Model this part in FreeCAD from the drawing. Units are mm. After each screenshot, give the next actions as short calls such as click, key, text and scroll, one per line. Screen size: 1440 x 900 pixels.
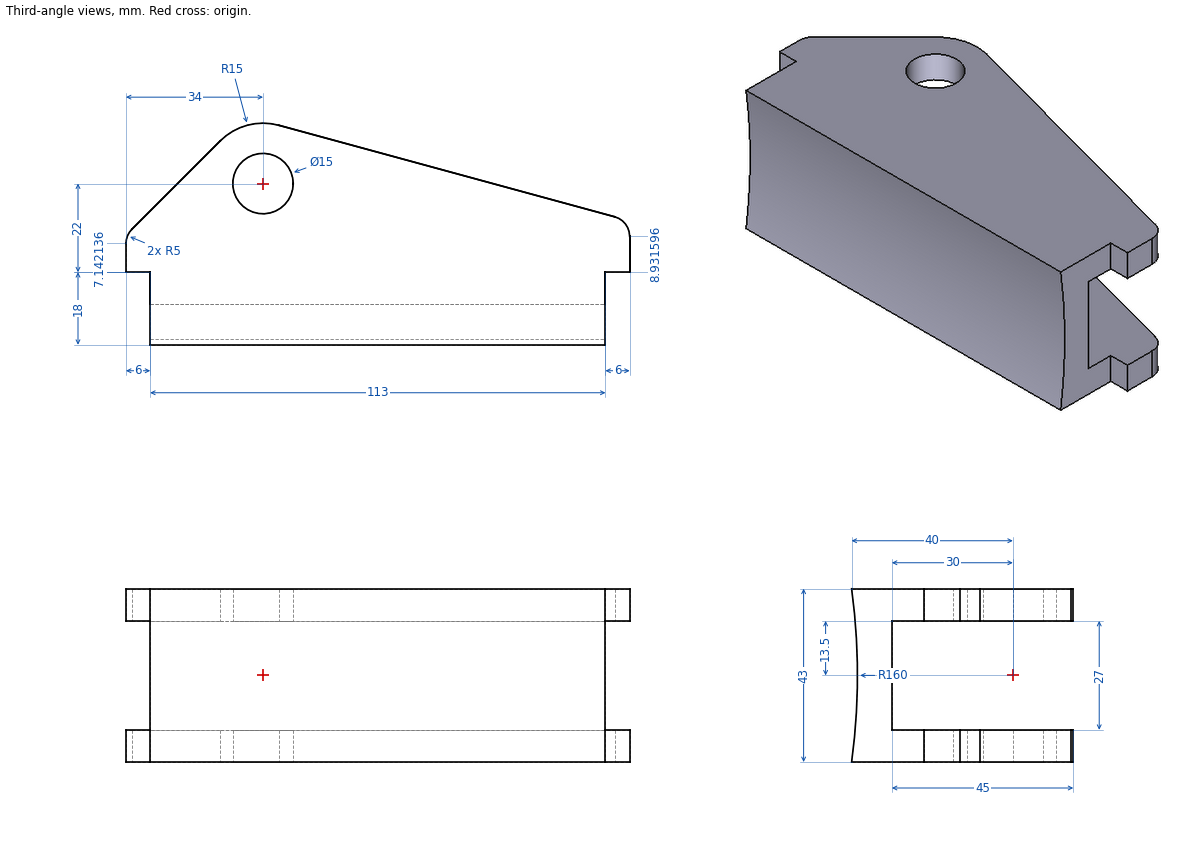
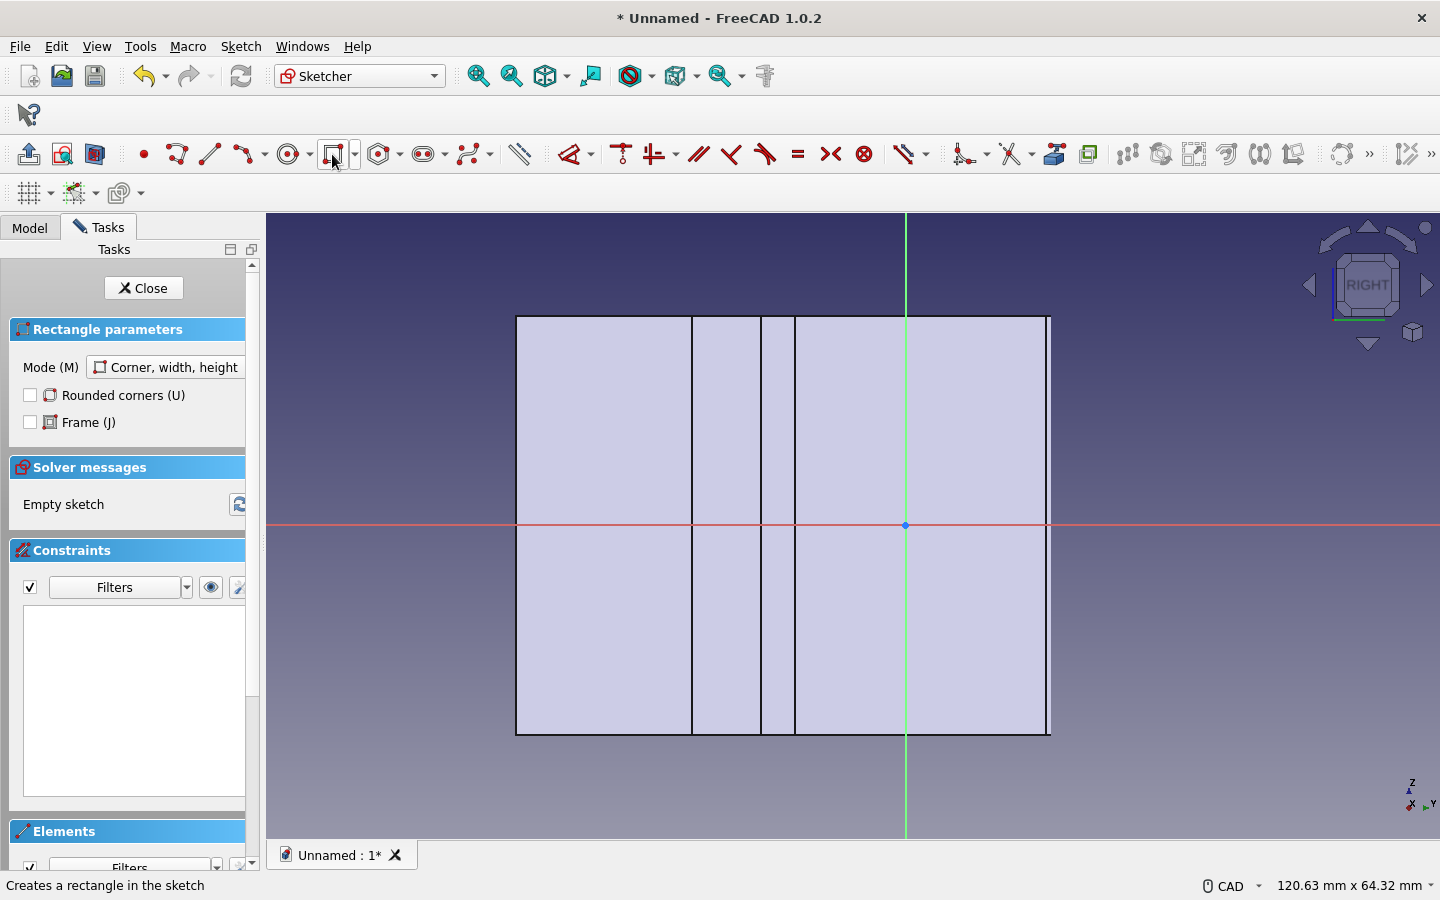
click(614, 394)
move(1052, 657)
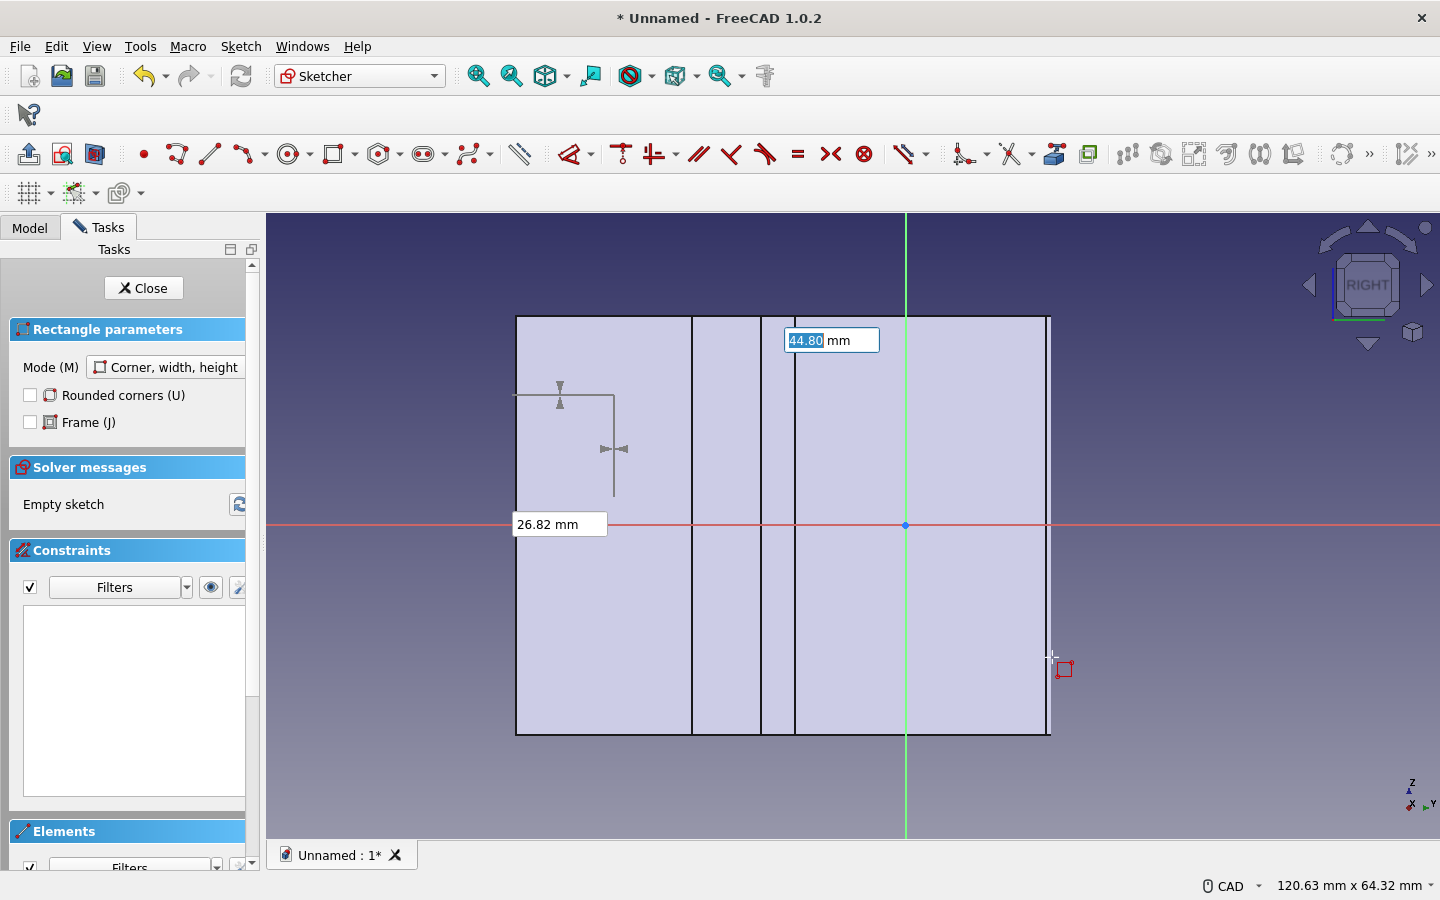
text(45)
key(Tab)
text(27)
key(Return)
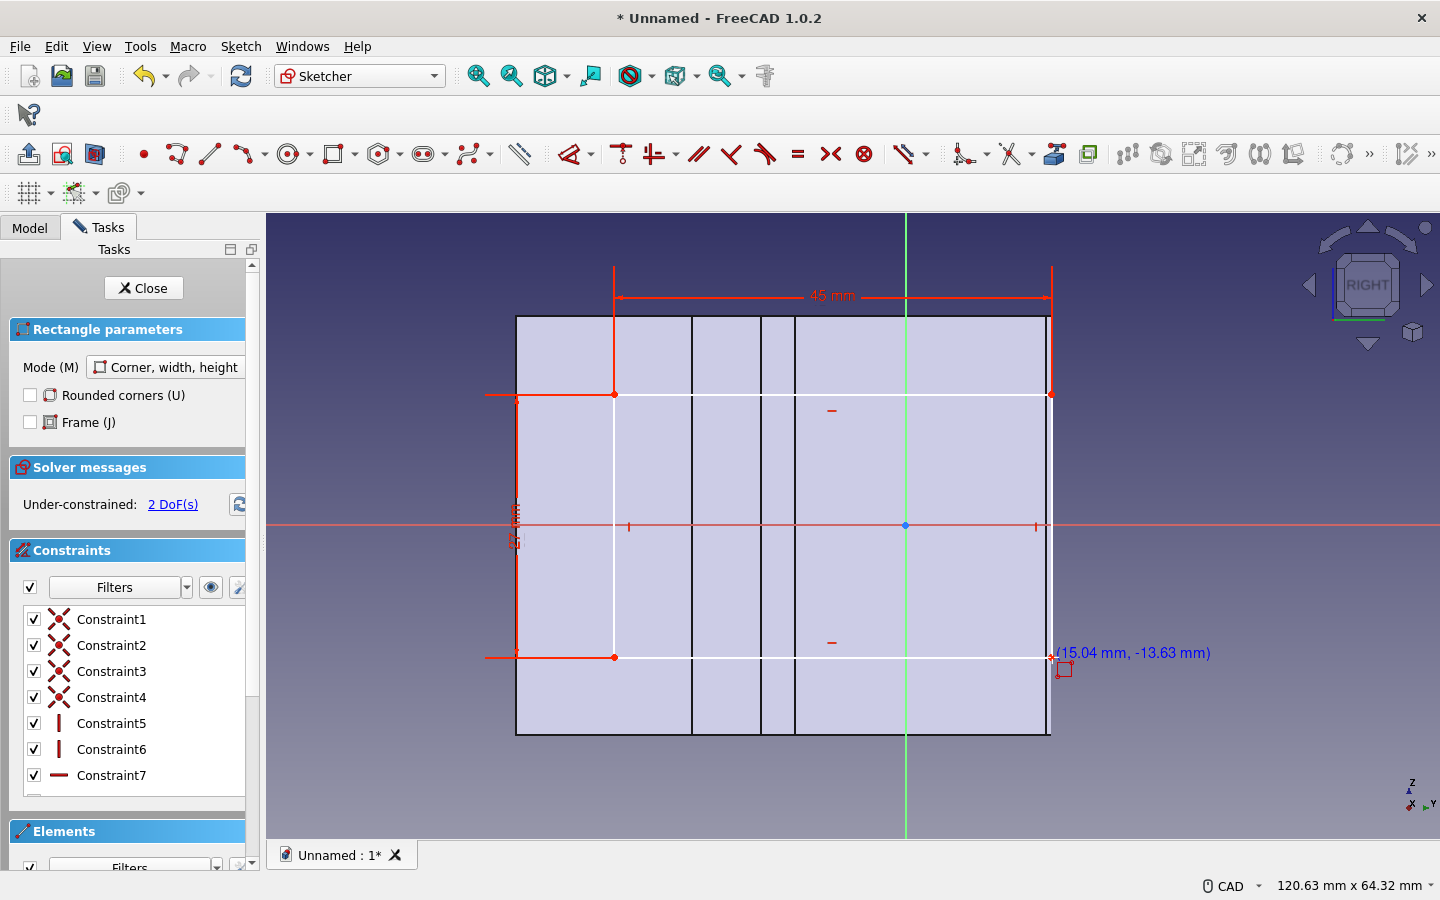
click(210, 154)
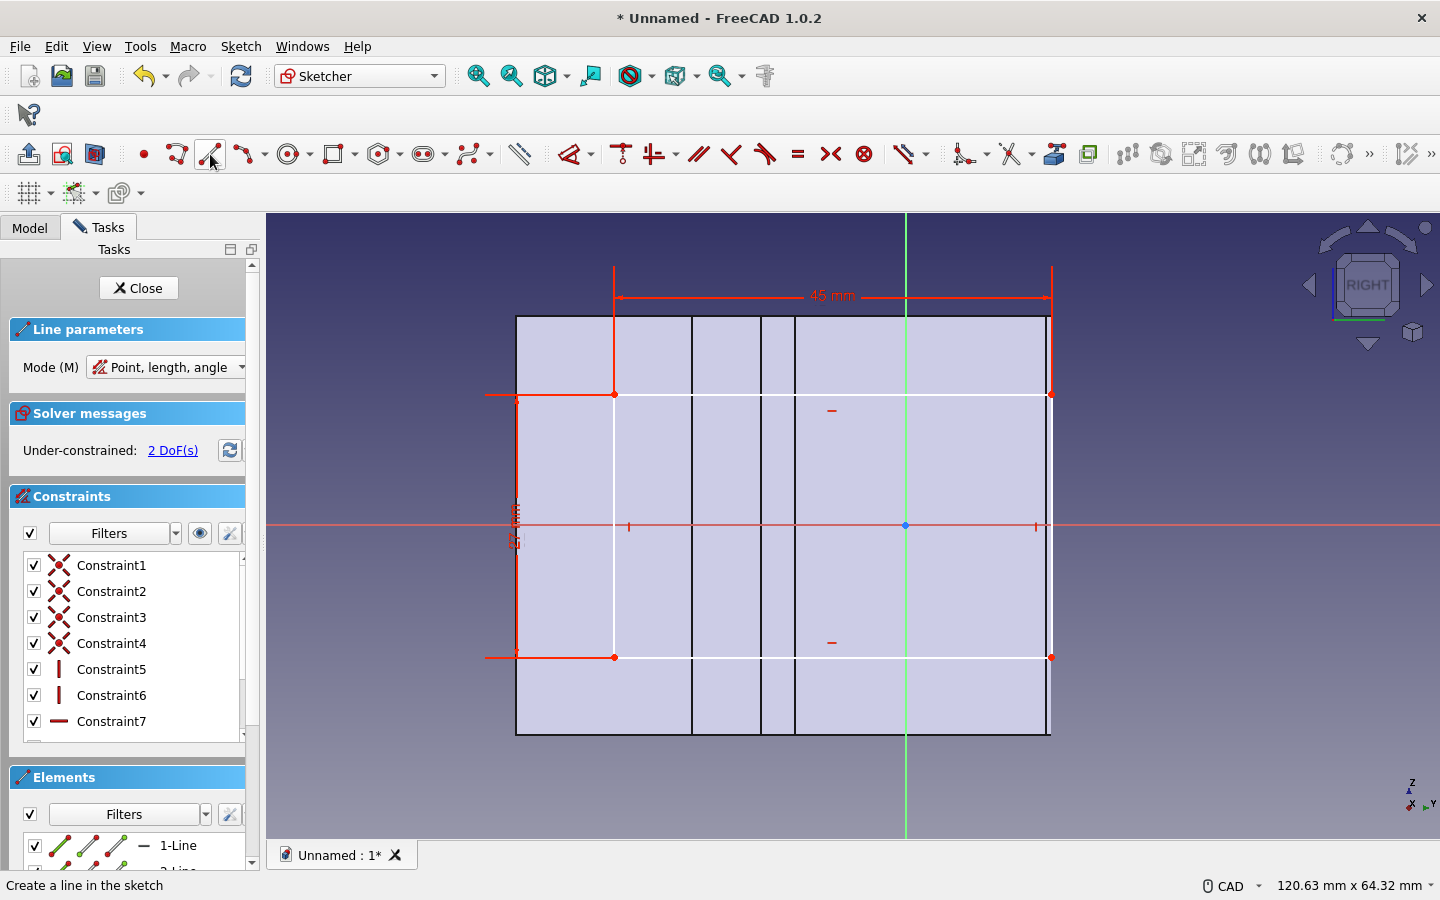
click(516, 316)
click(516, 735)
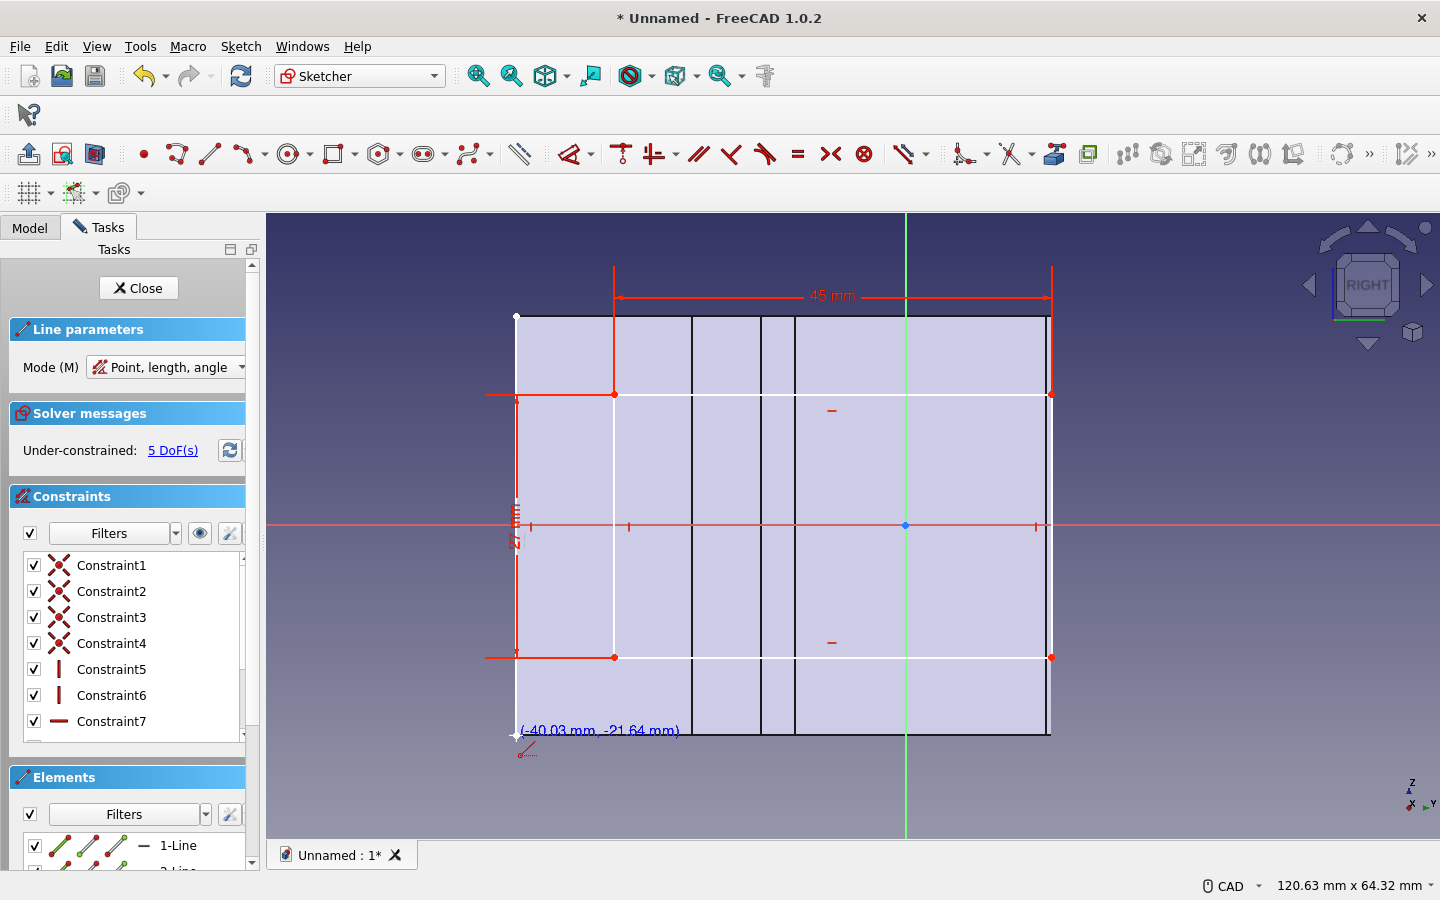
click(242, 154)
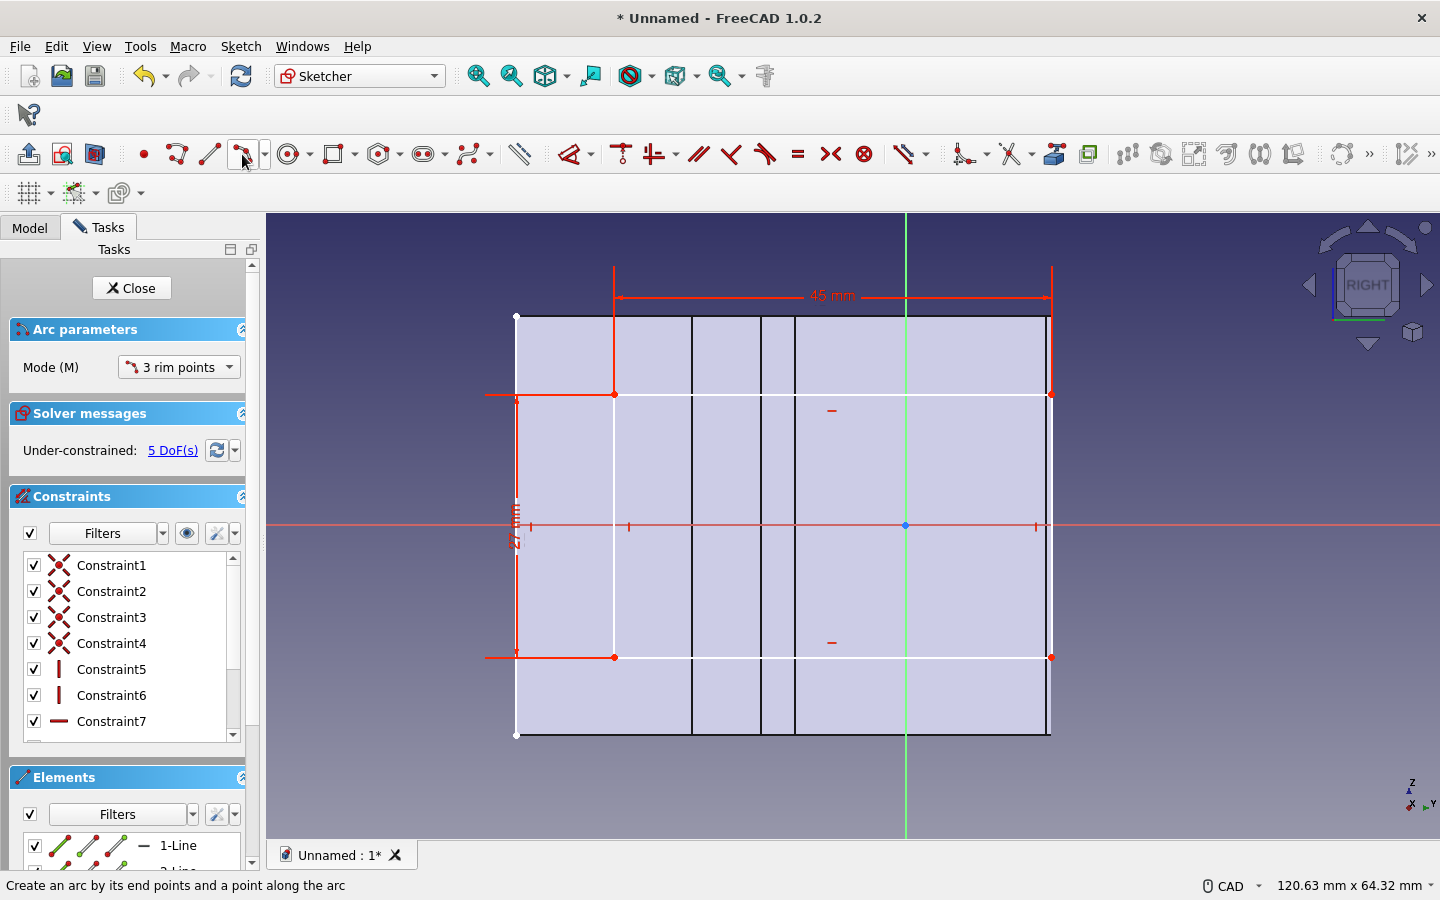
click(516, 736)
click(516, 317)
click(530, 567)
key(Escape)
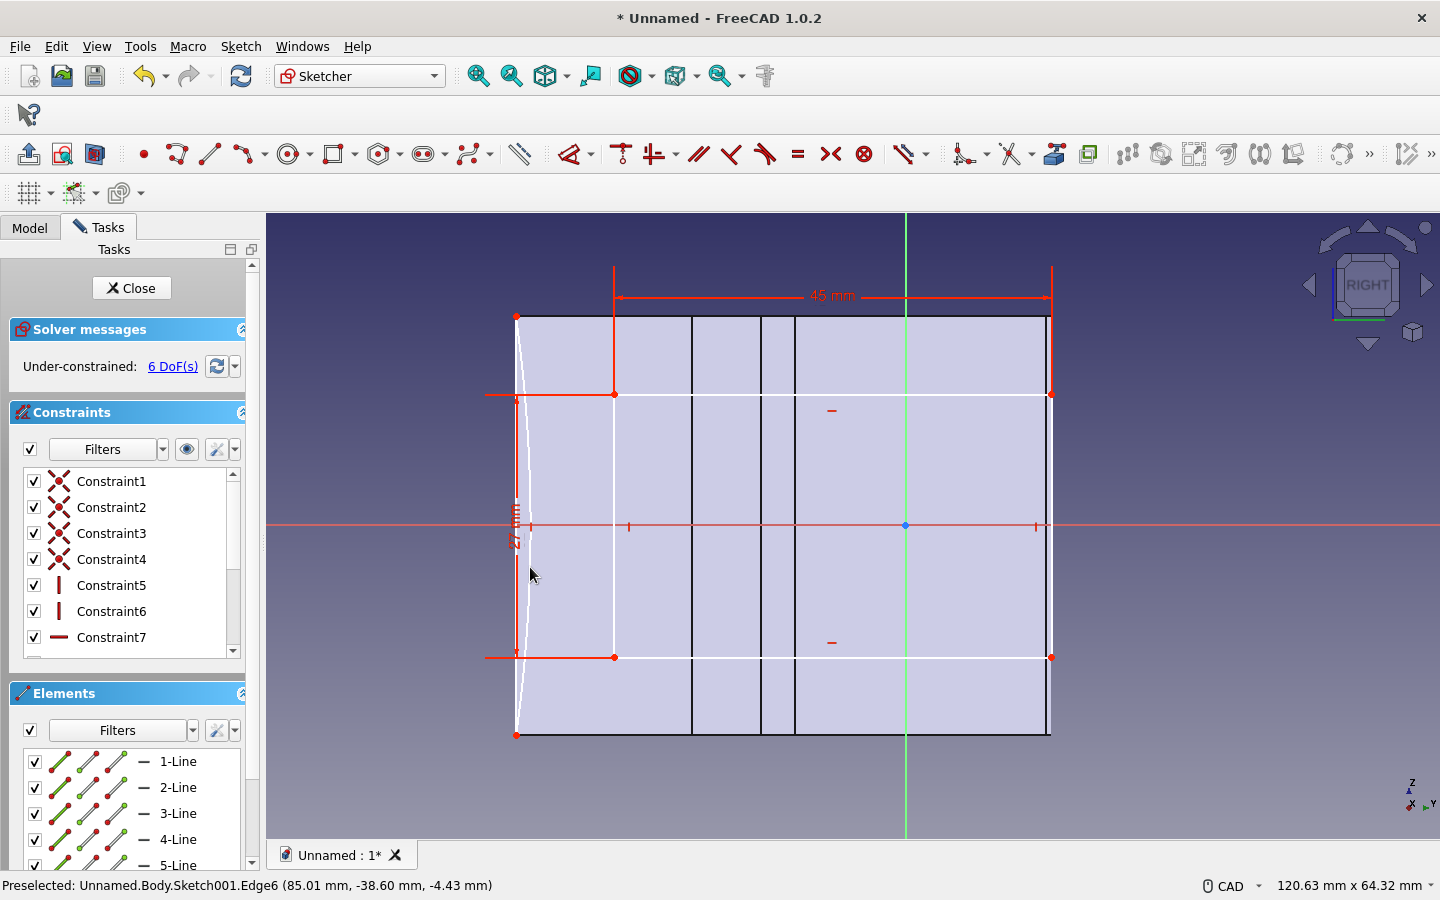
scroll(1221, 526, down, 5)